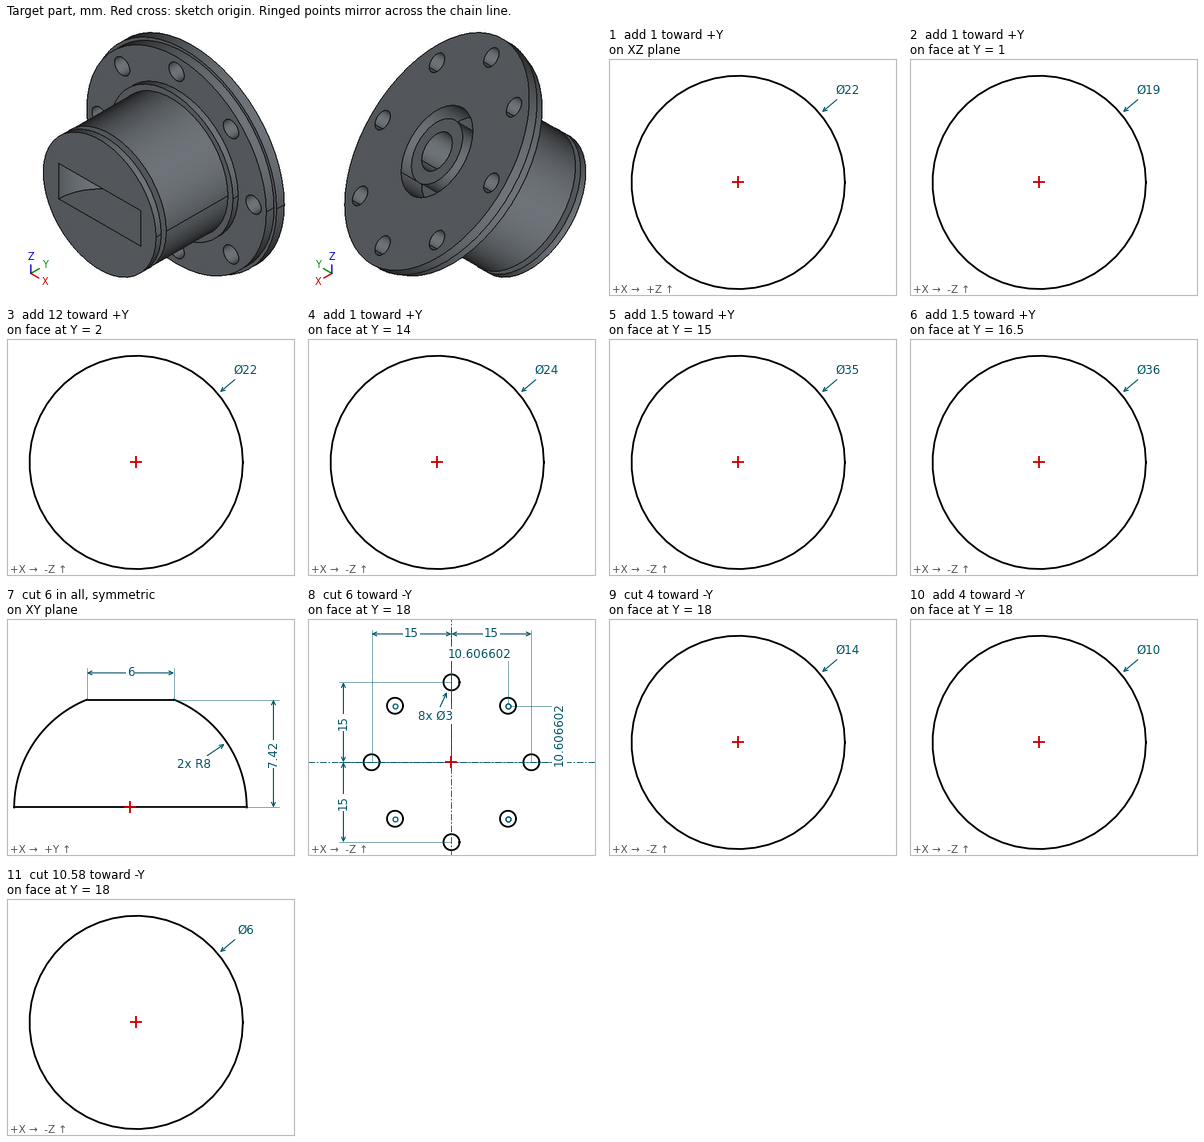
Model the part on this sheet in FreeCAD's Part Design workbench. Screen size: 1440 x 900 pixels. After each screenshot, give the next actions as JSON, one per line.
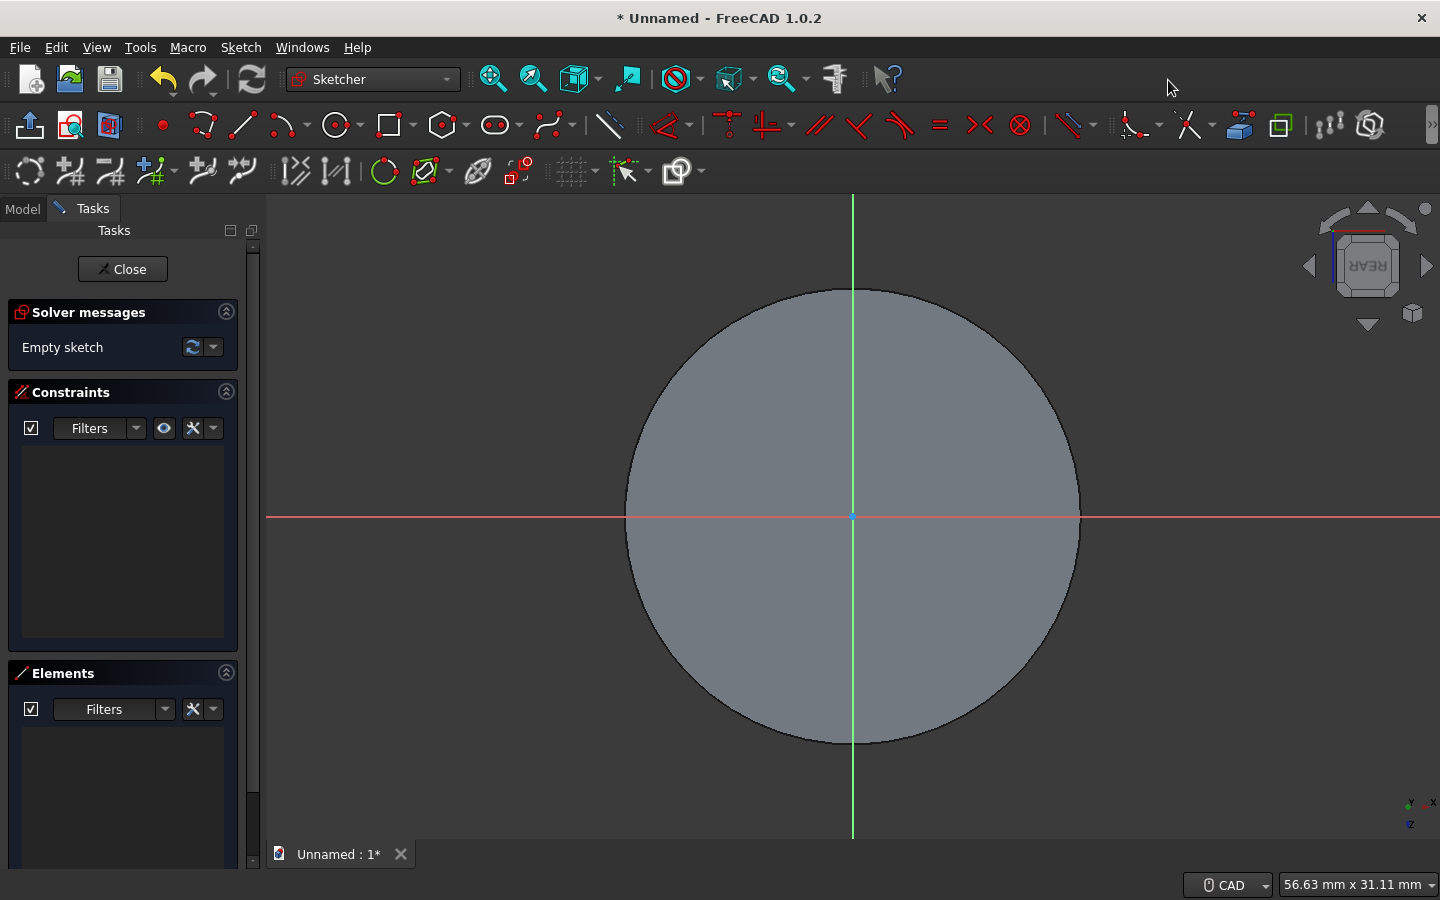
{"action": "left_click", "coordinate": [336, 126]}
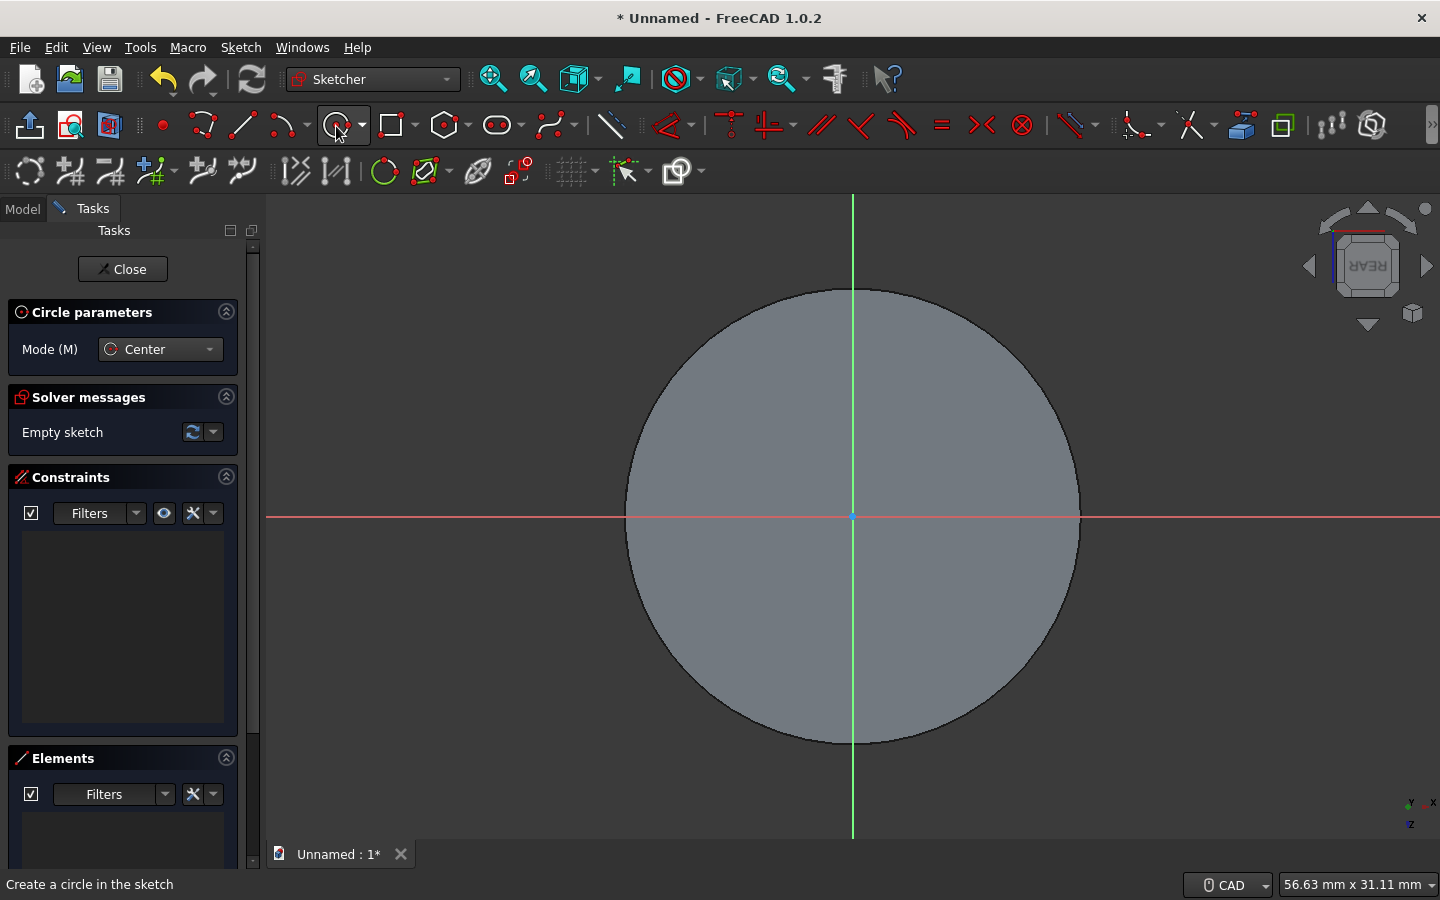
{"action": "left_click", "coordinate": [853, 516]}
{"action": "mouse_move", "coordinate": [1029, 341]}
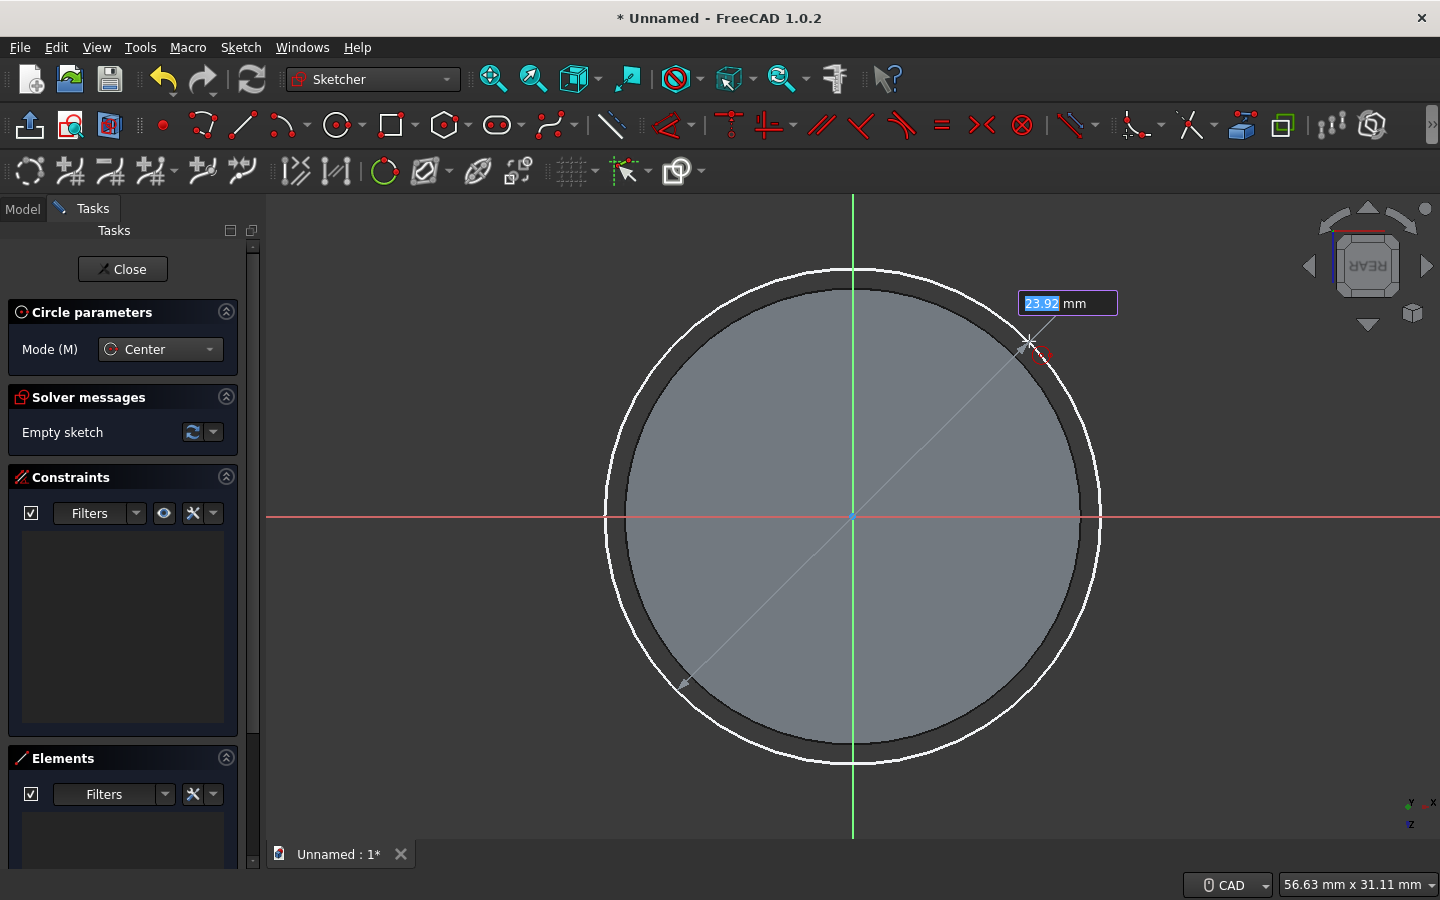
{"action": "type", "text": "24"}
{"action": "key", "text": "Return"}
{"action": "key", "text": "Escape"}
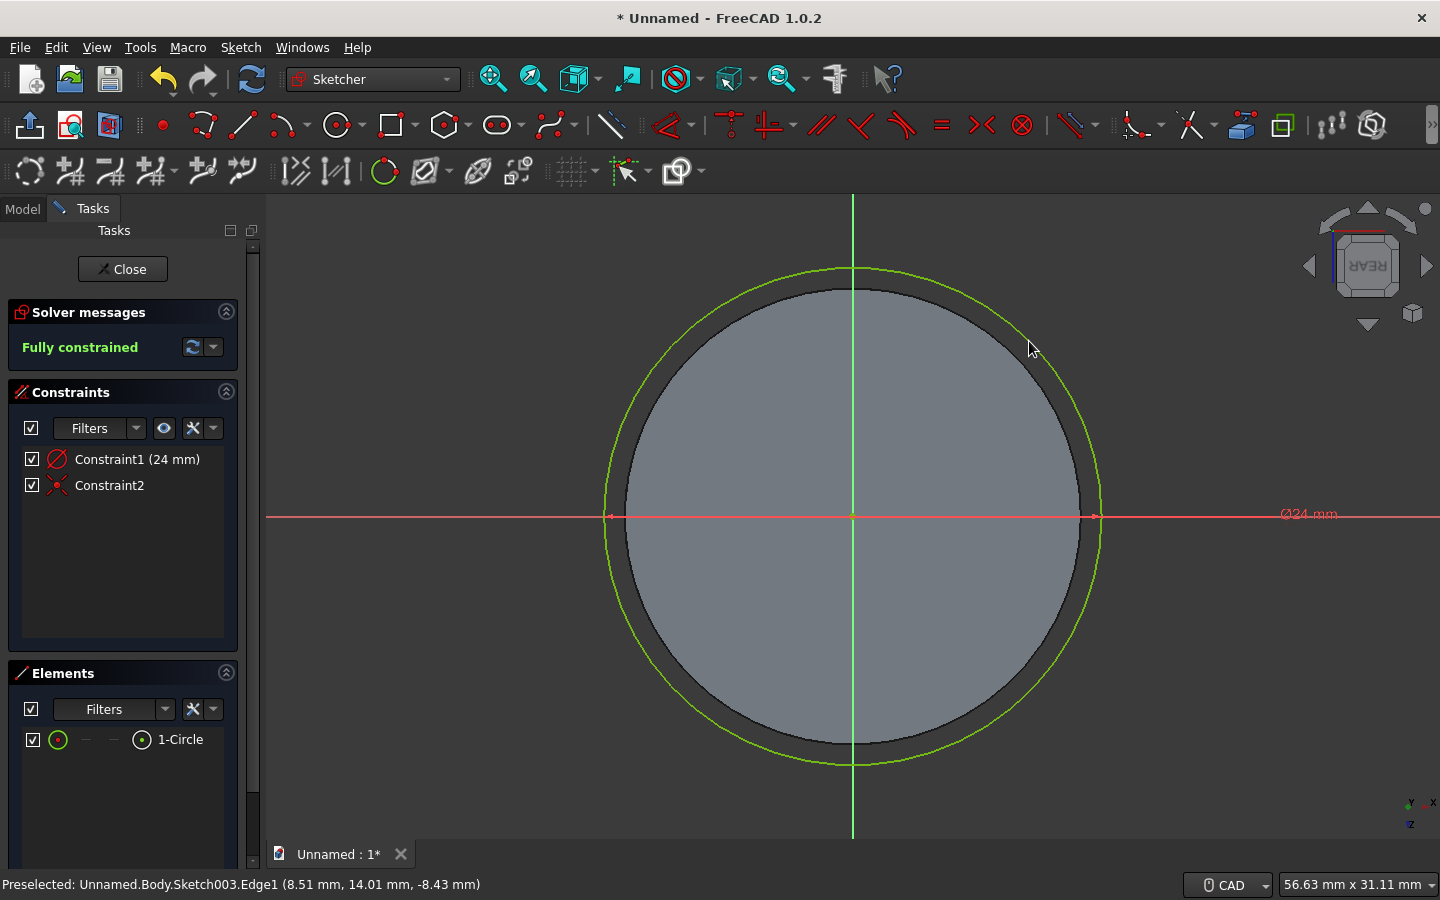
{"action": "left_click", "coordinate": [123, 269]}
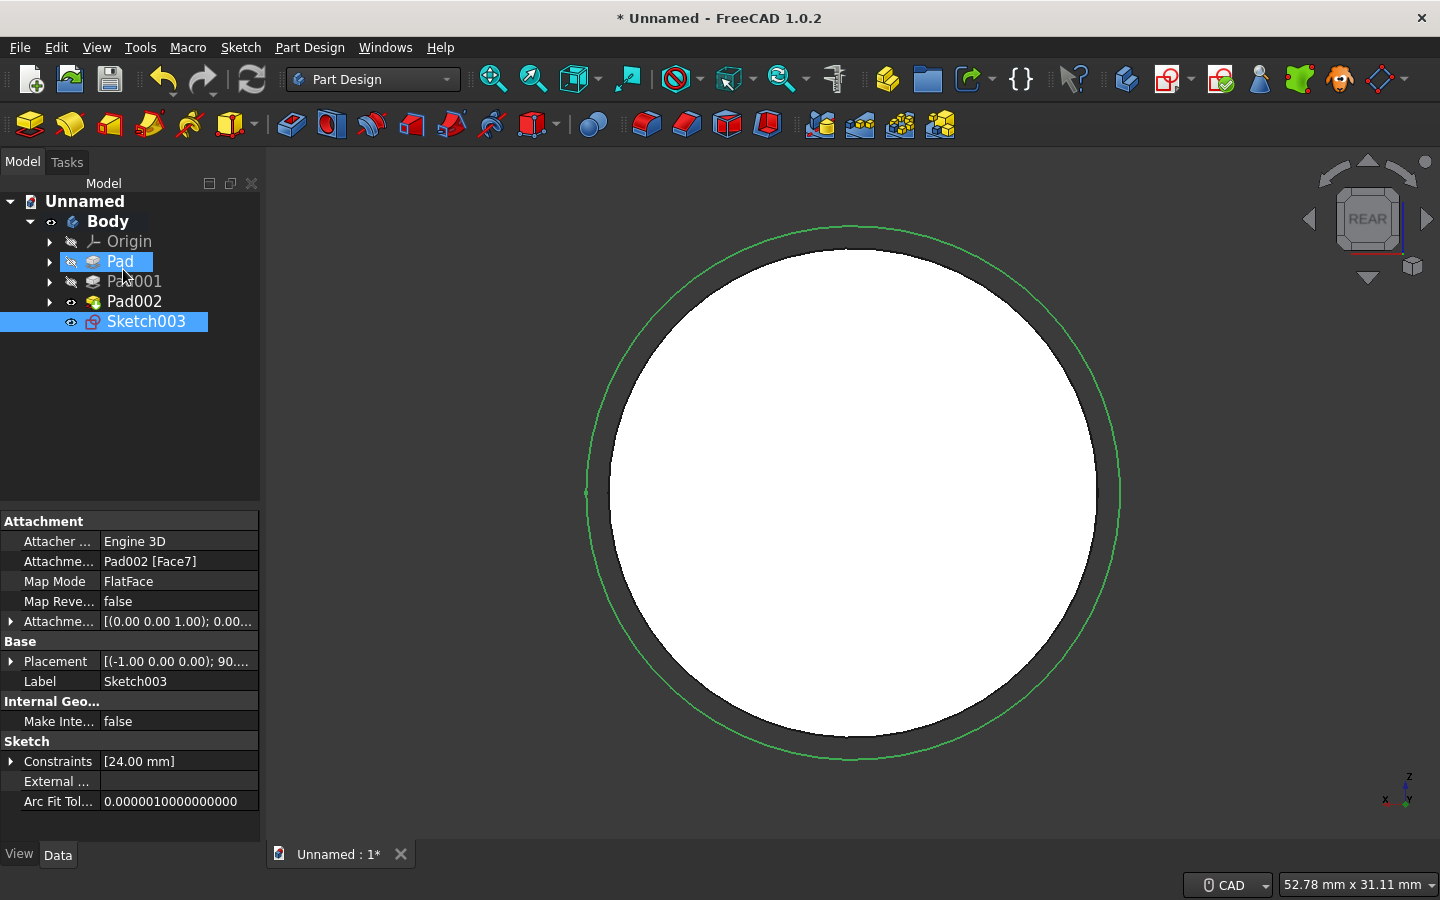
{"action": "left_click", "coordinate": [30, 124]}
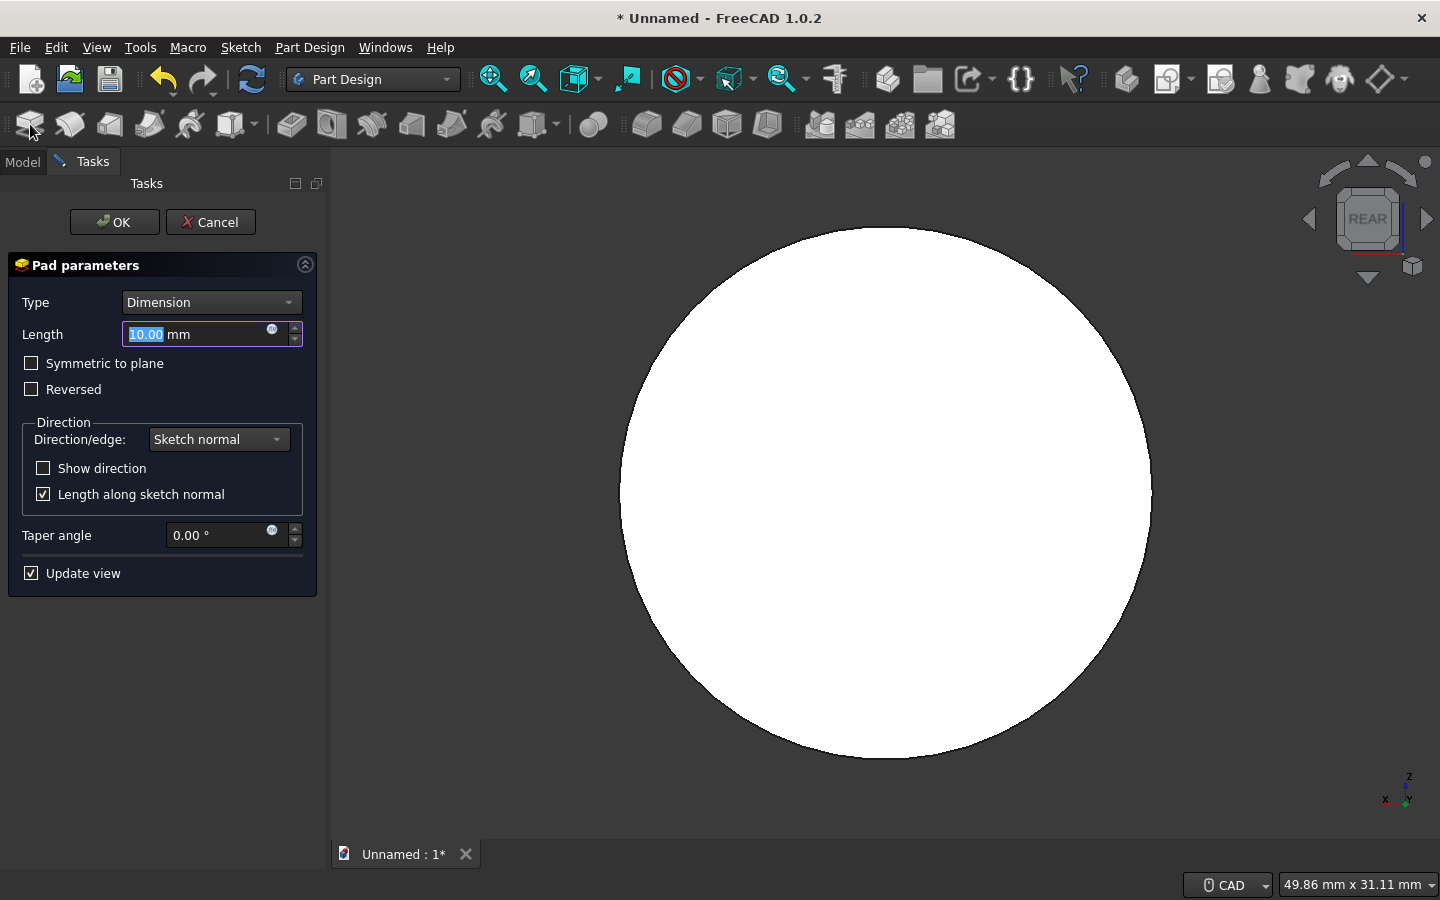
{"action": "type", "text": "1"}
{"action": "key", "text": "Tab"}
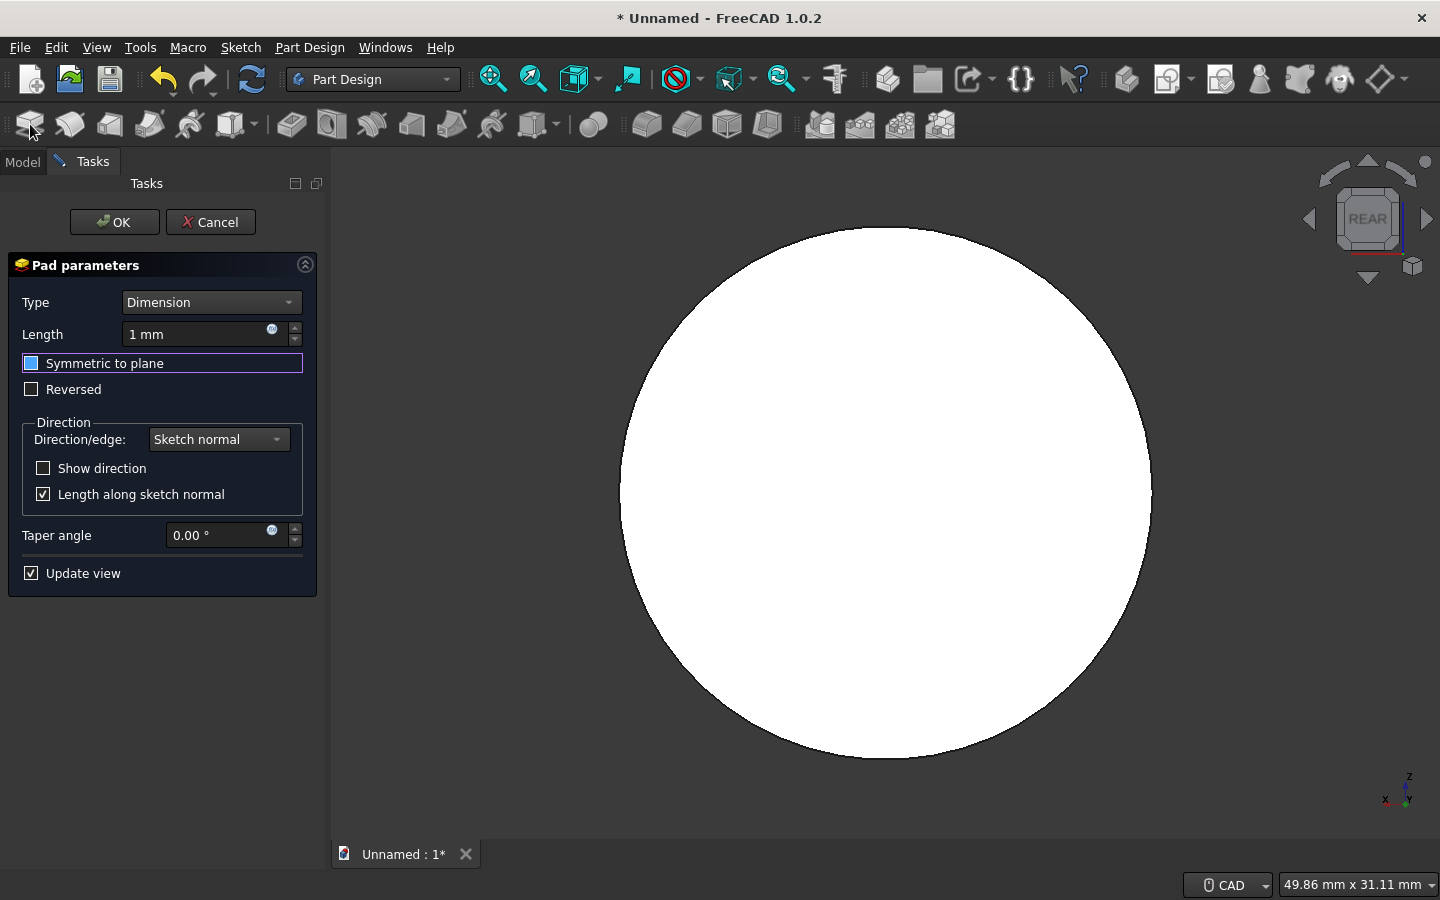
{"action": "left_click", "coordinate": [115, 222]}